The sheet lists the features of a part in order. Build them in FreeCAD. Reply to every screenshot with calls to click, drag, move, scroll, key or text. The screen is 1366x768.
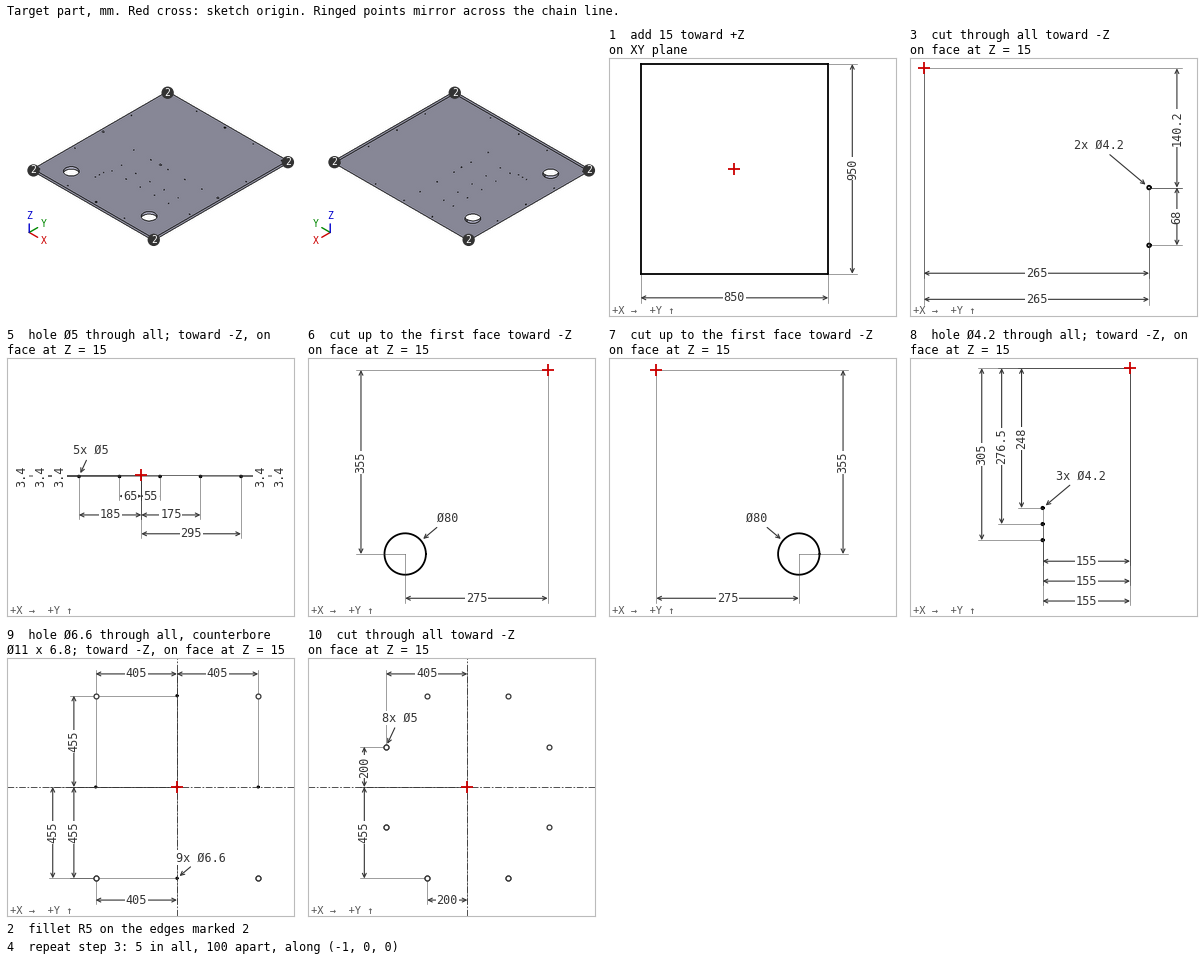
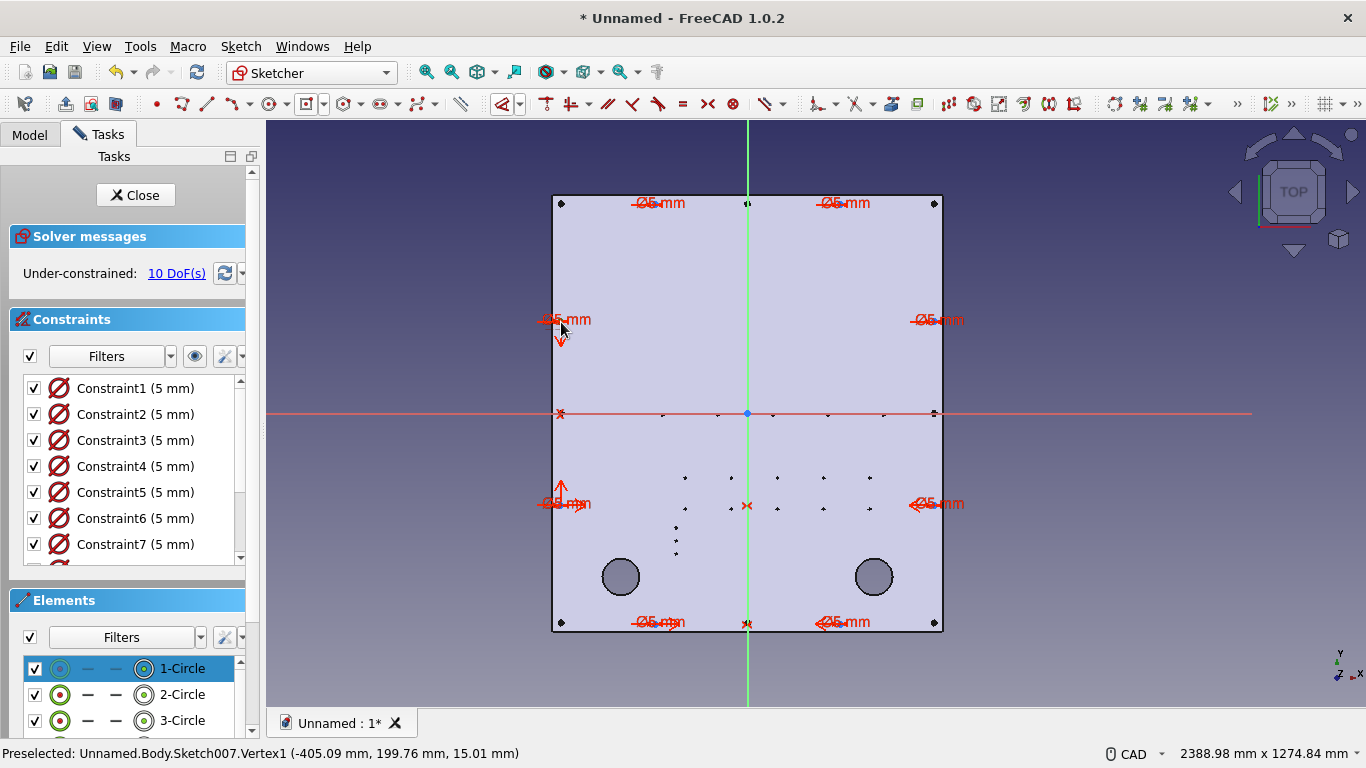
click(934, 322)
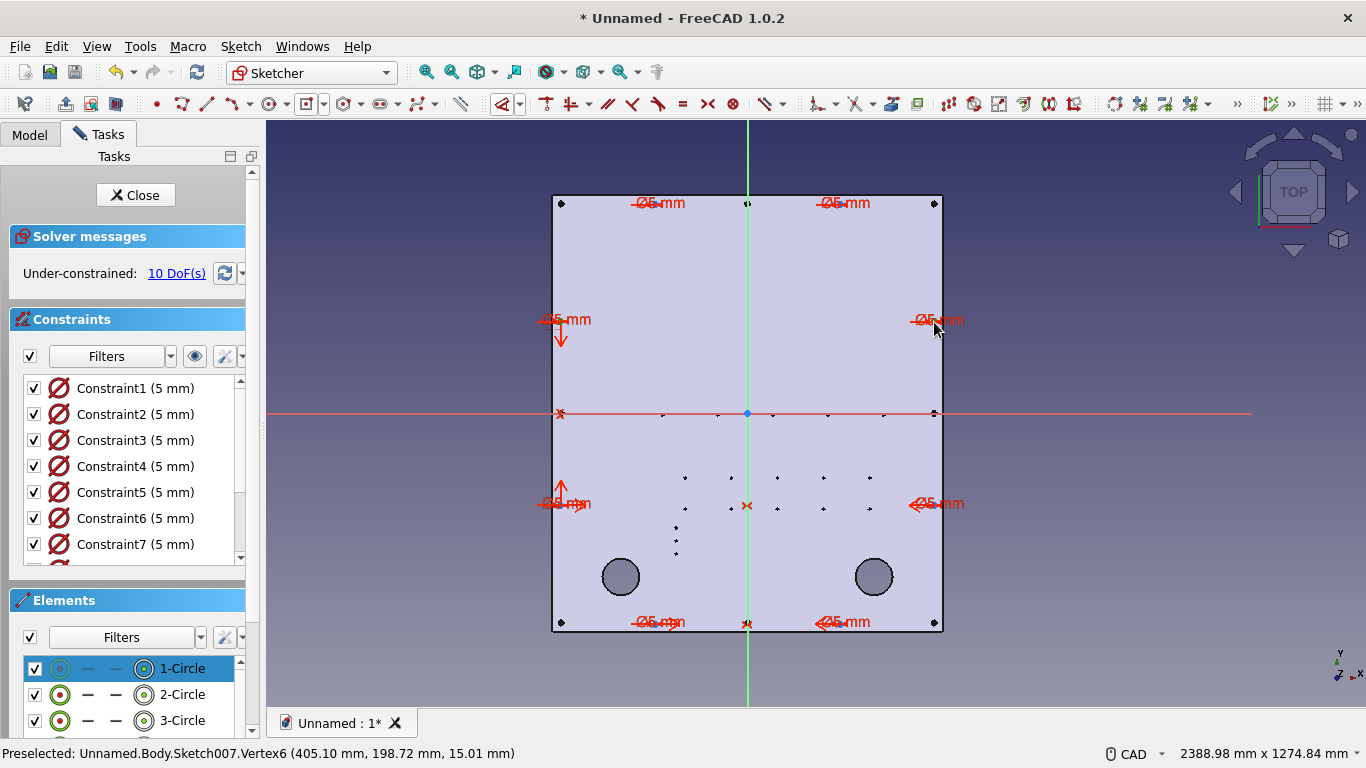
click(748, 641)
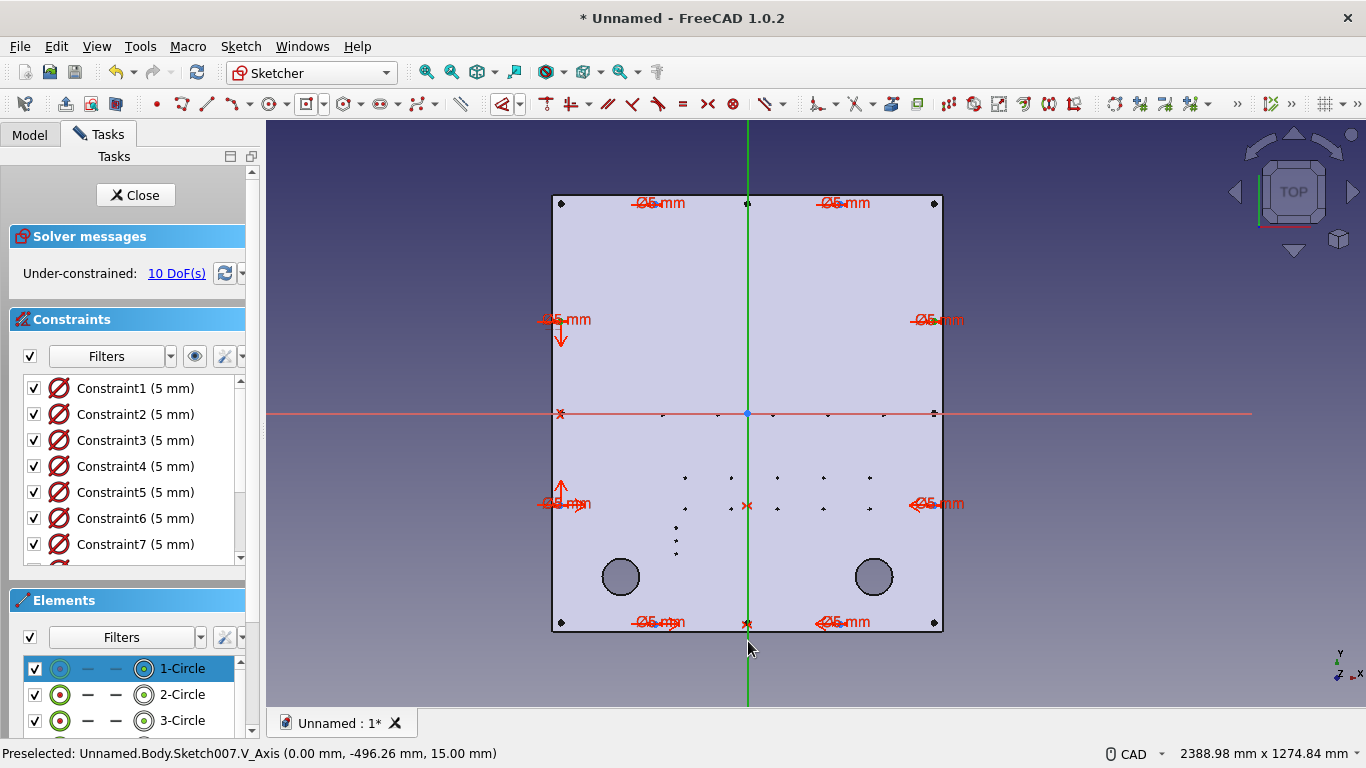
click(708, 104)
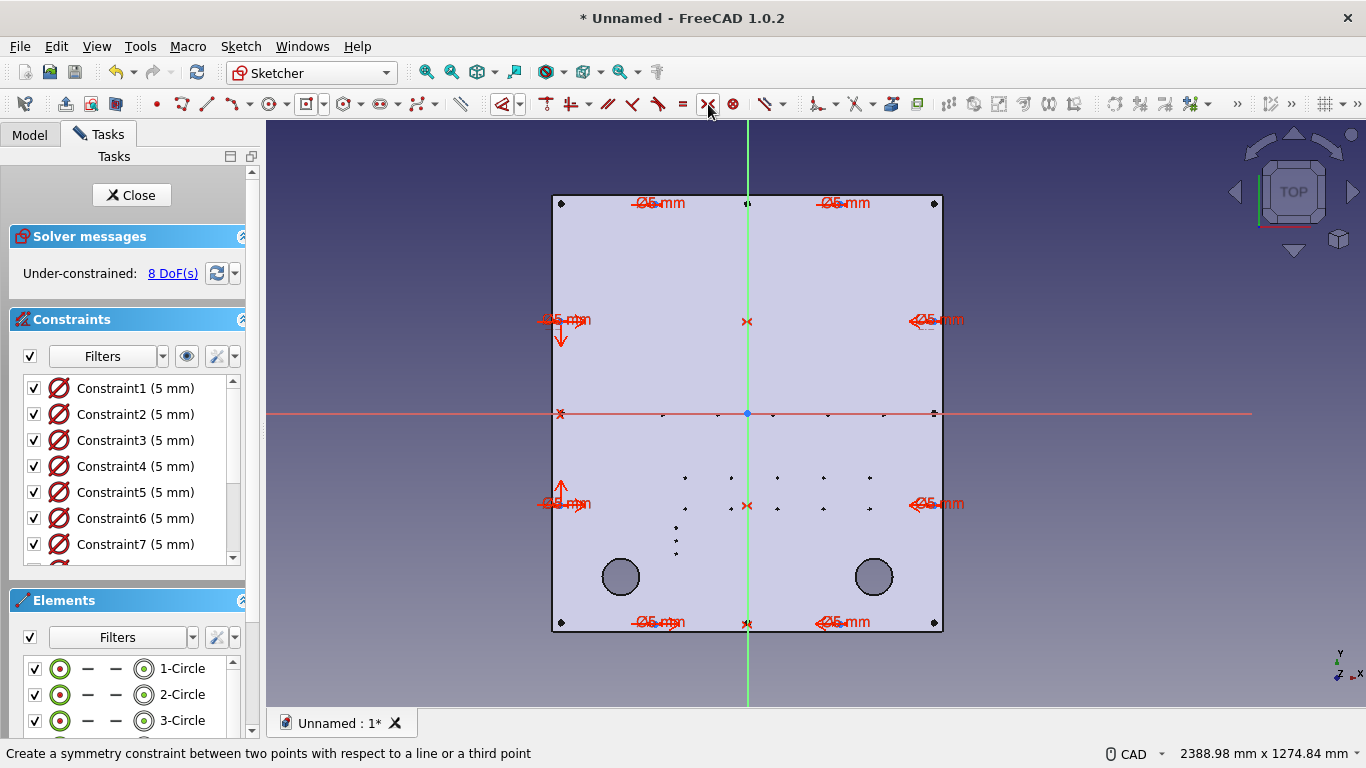
click(840, 624)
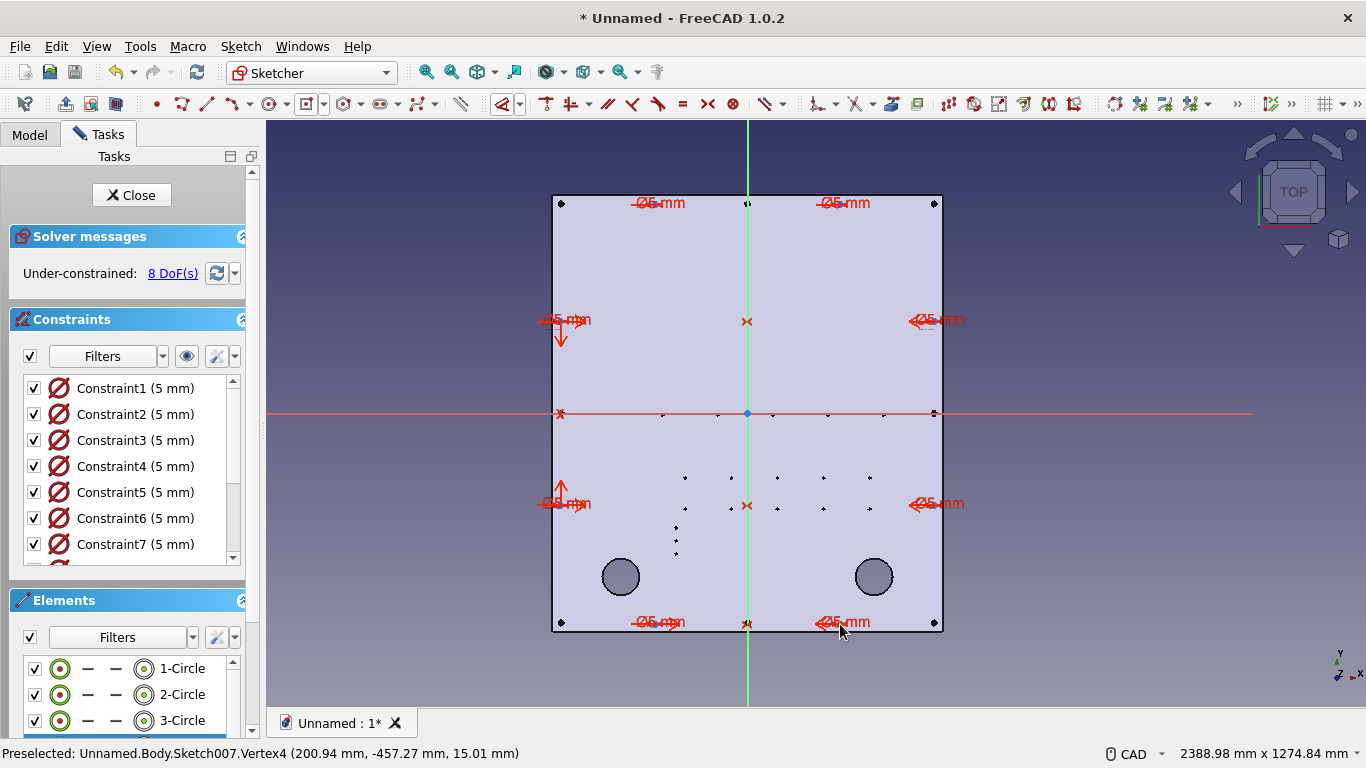
click(840, 205)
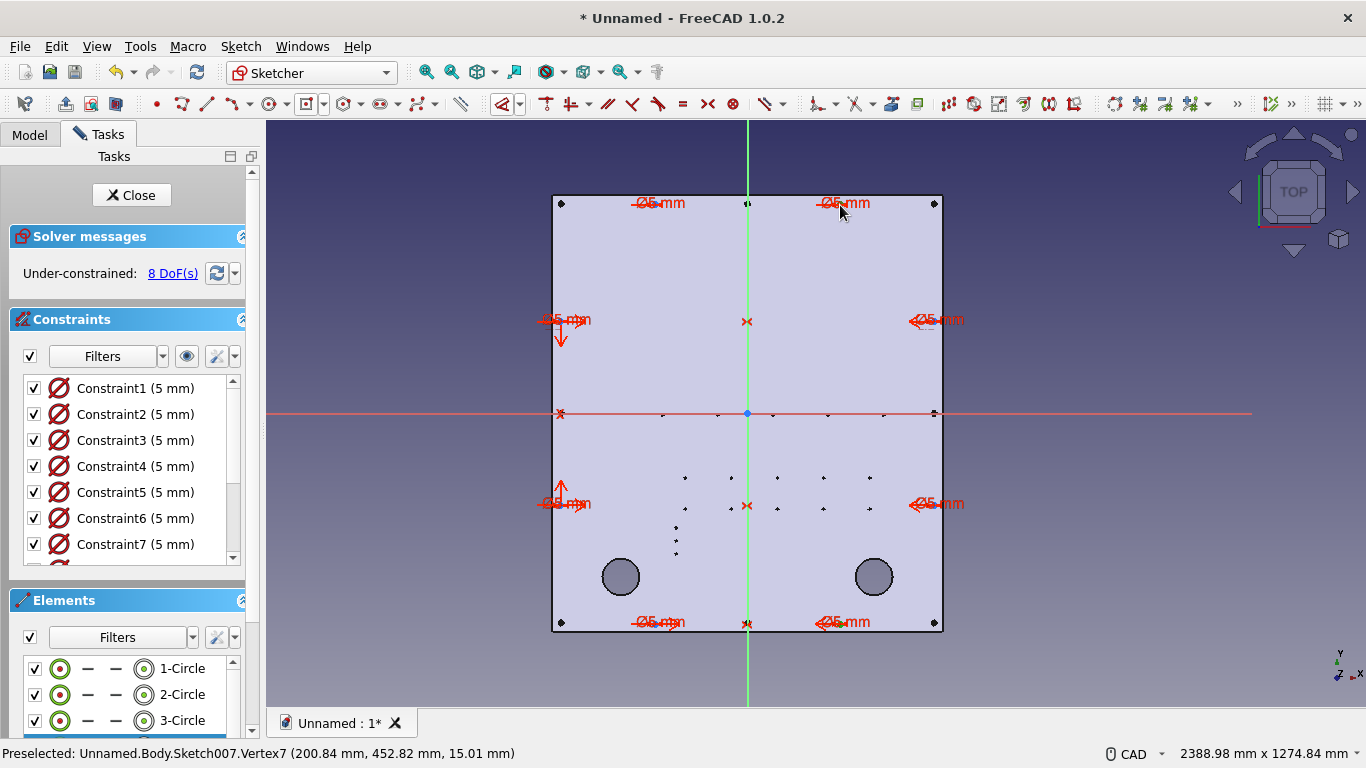
click(359, 413)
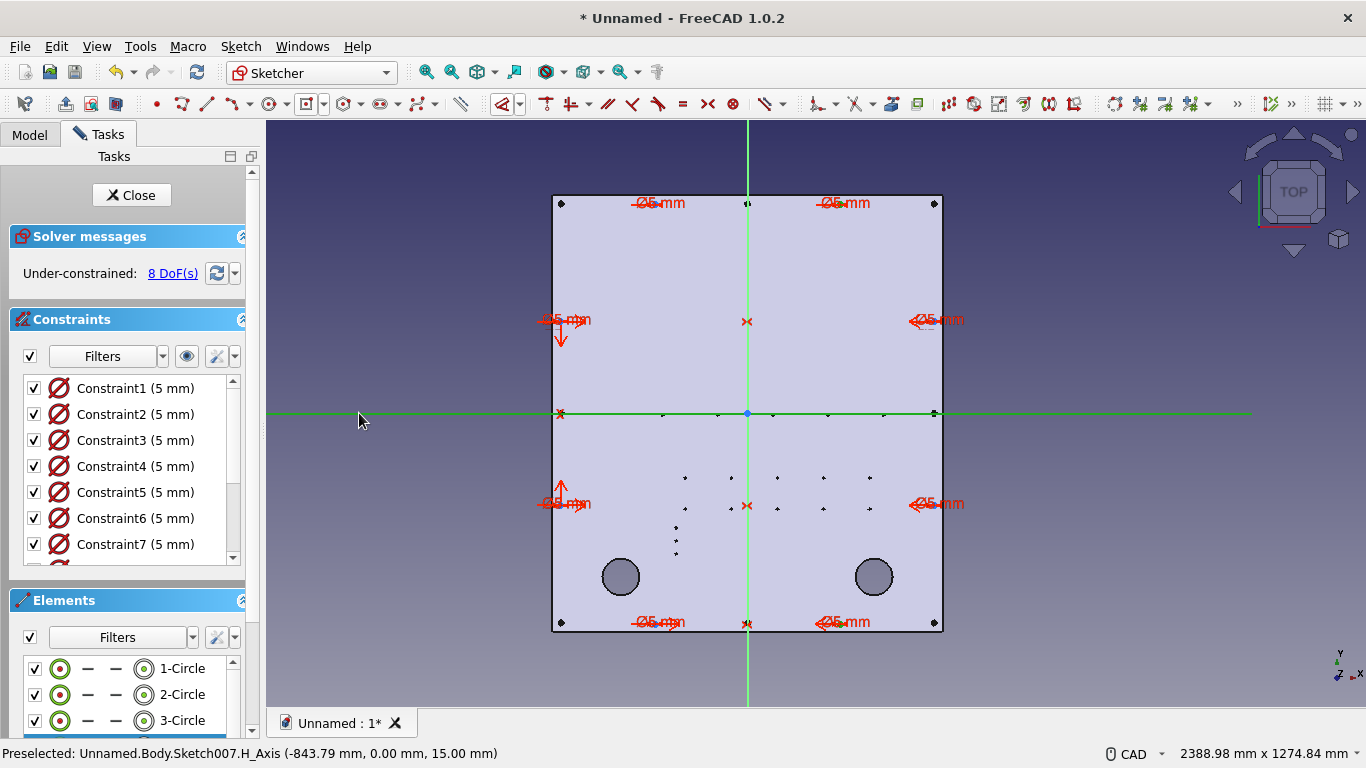
click(708, 104)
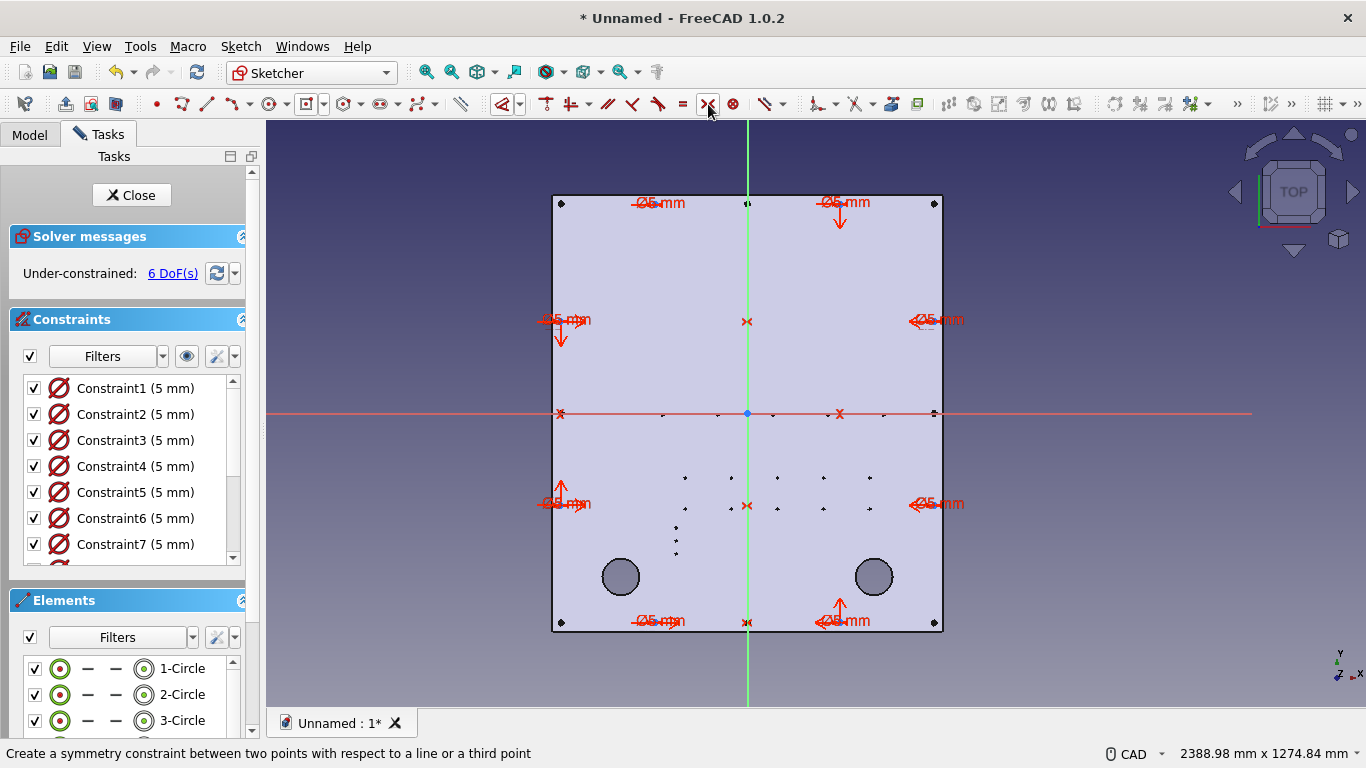
click(655, 623)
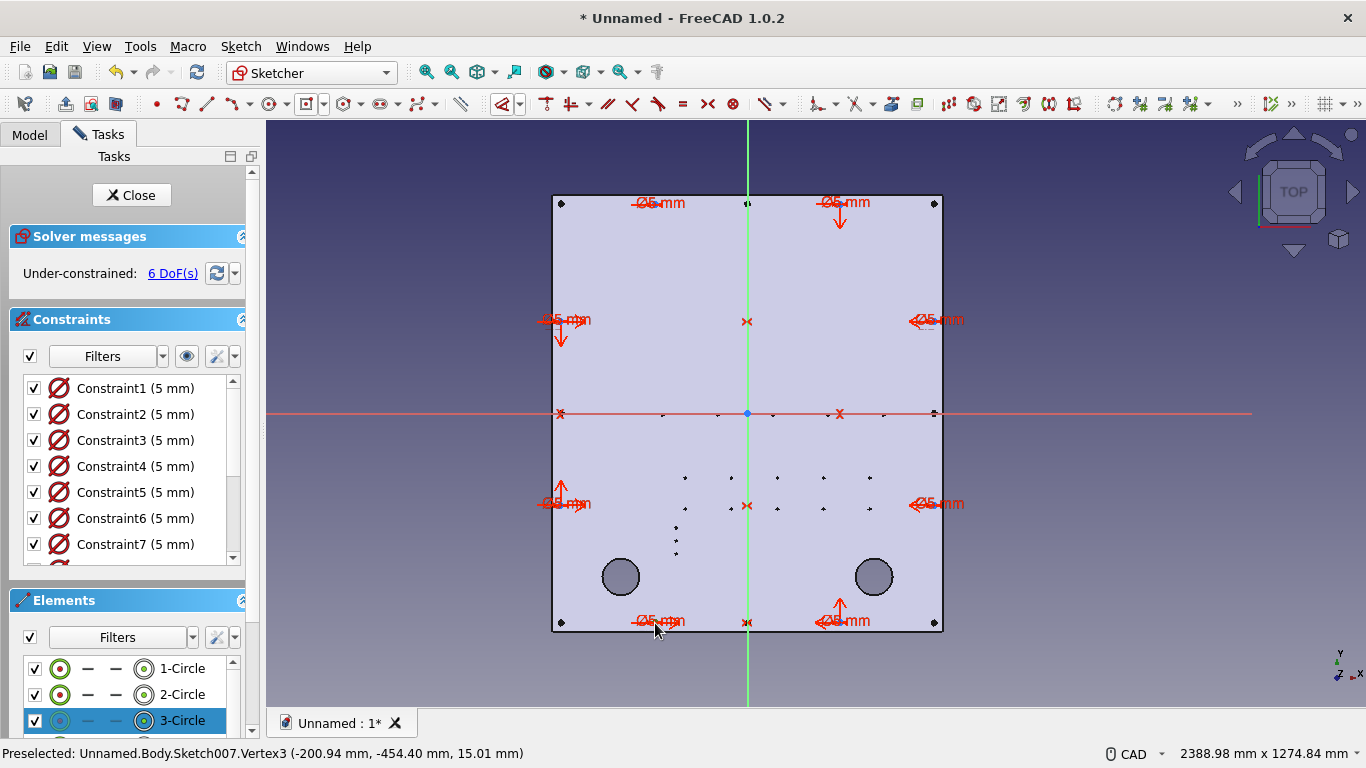
click(655, 205)